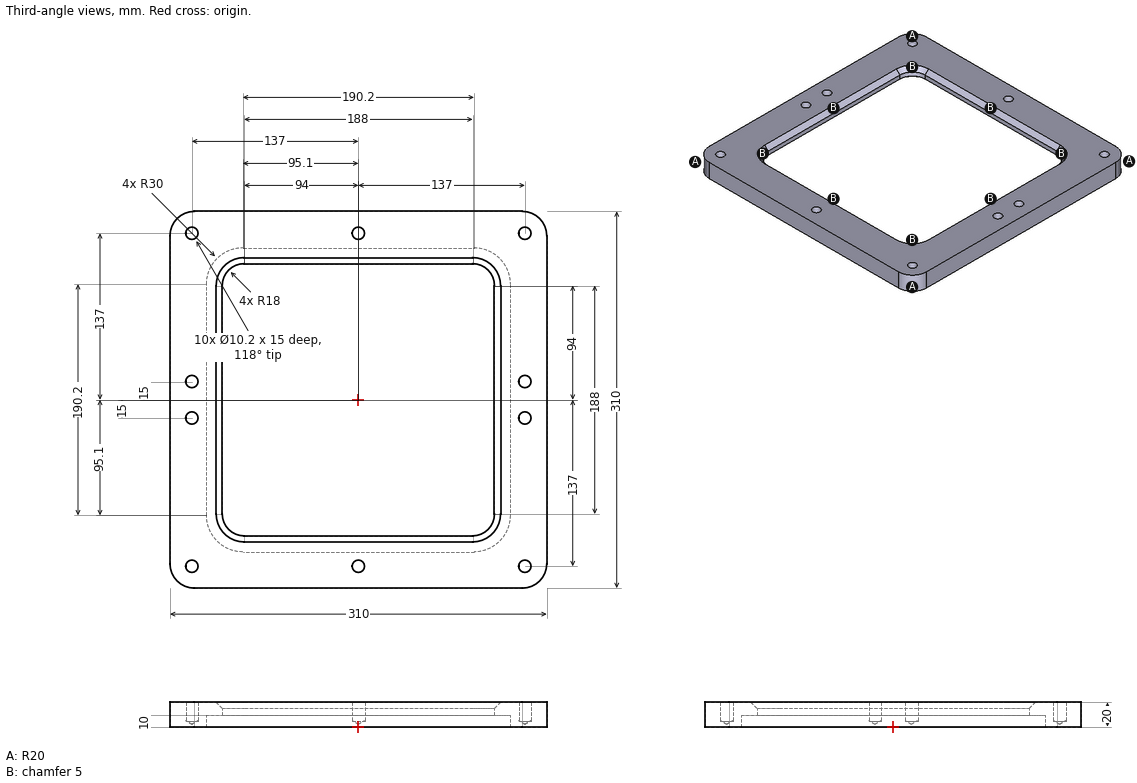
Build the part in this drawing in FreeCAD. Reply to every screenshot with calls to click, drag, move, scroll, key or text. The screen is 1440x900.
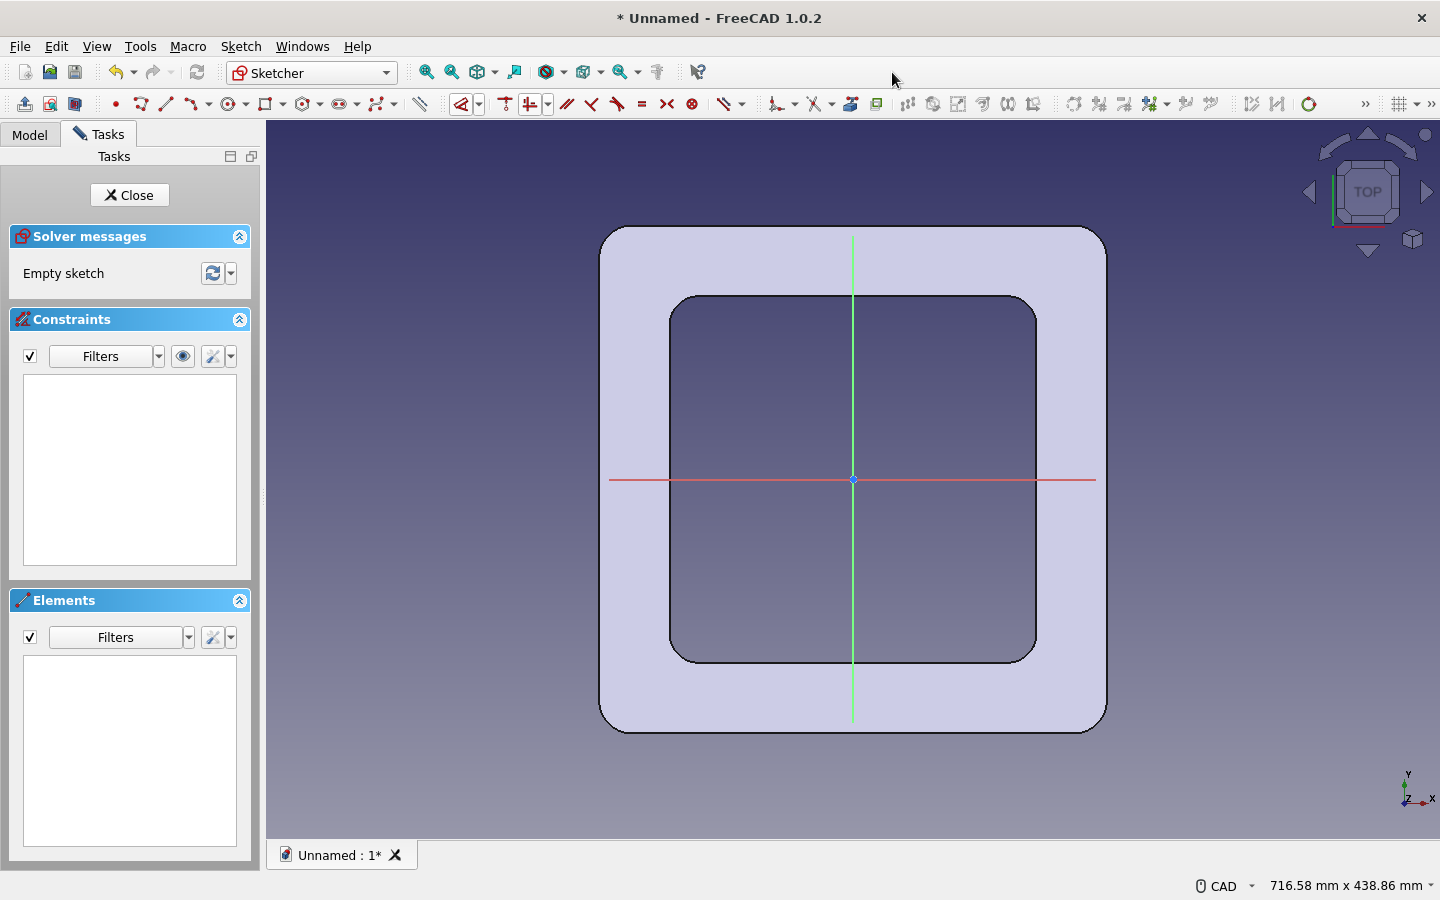
click(228, 104)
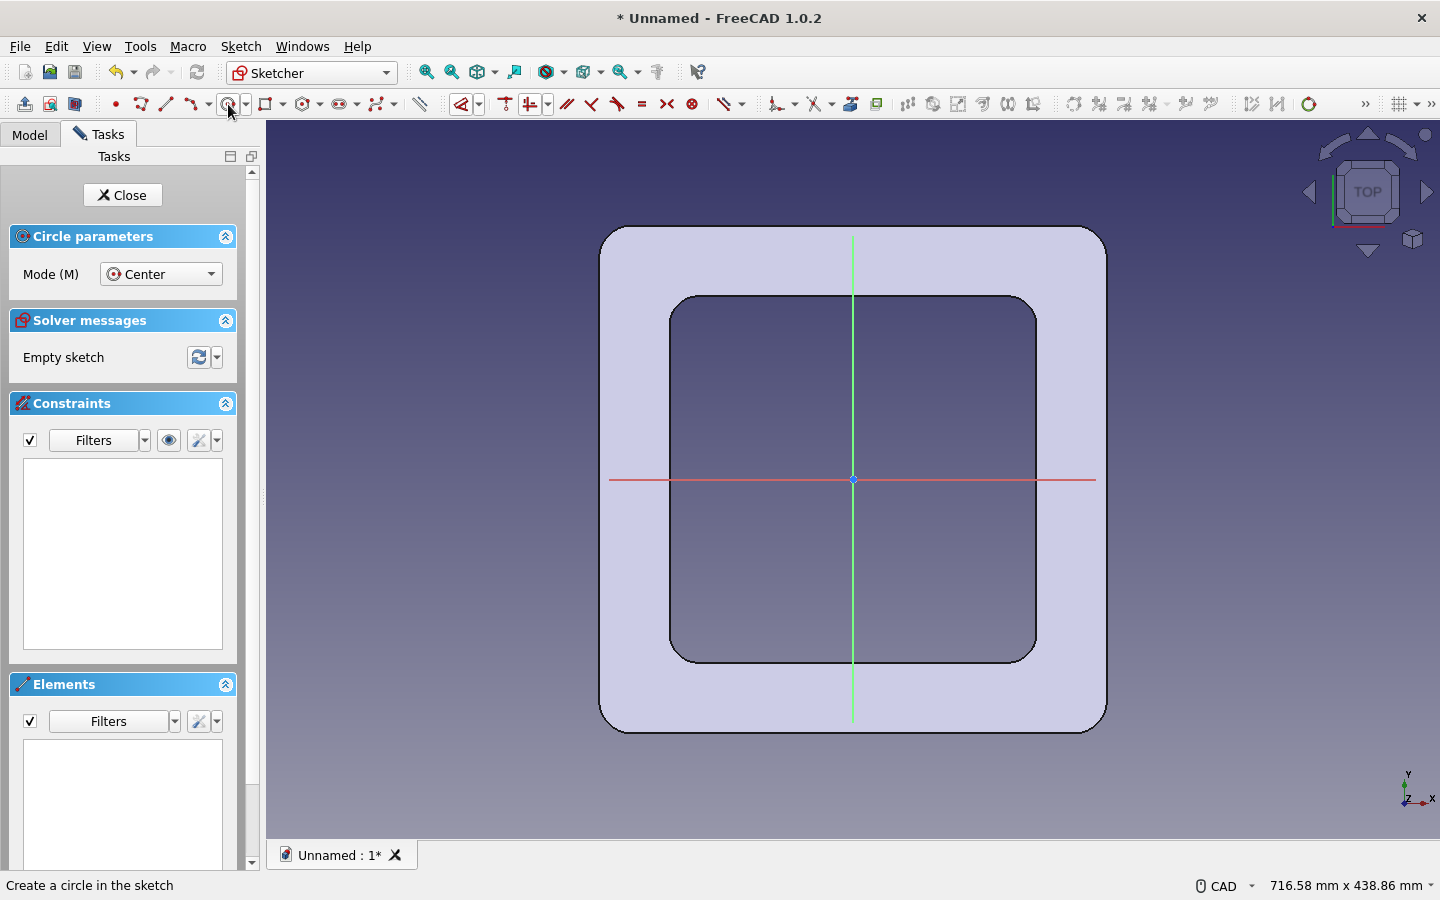
scroll(629, 255, up, 5)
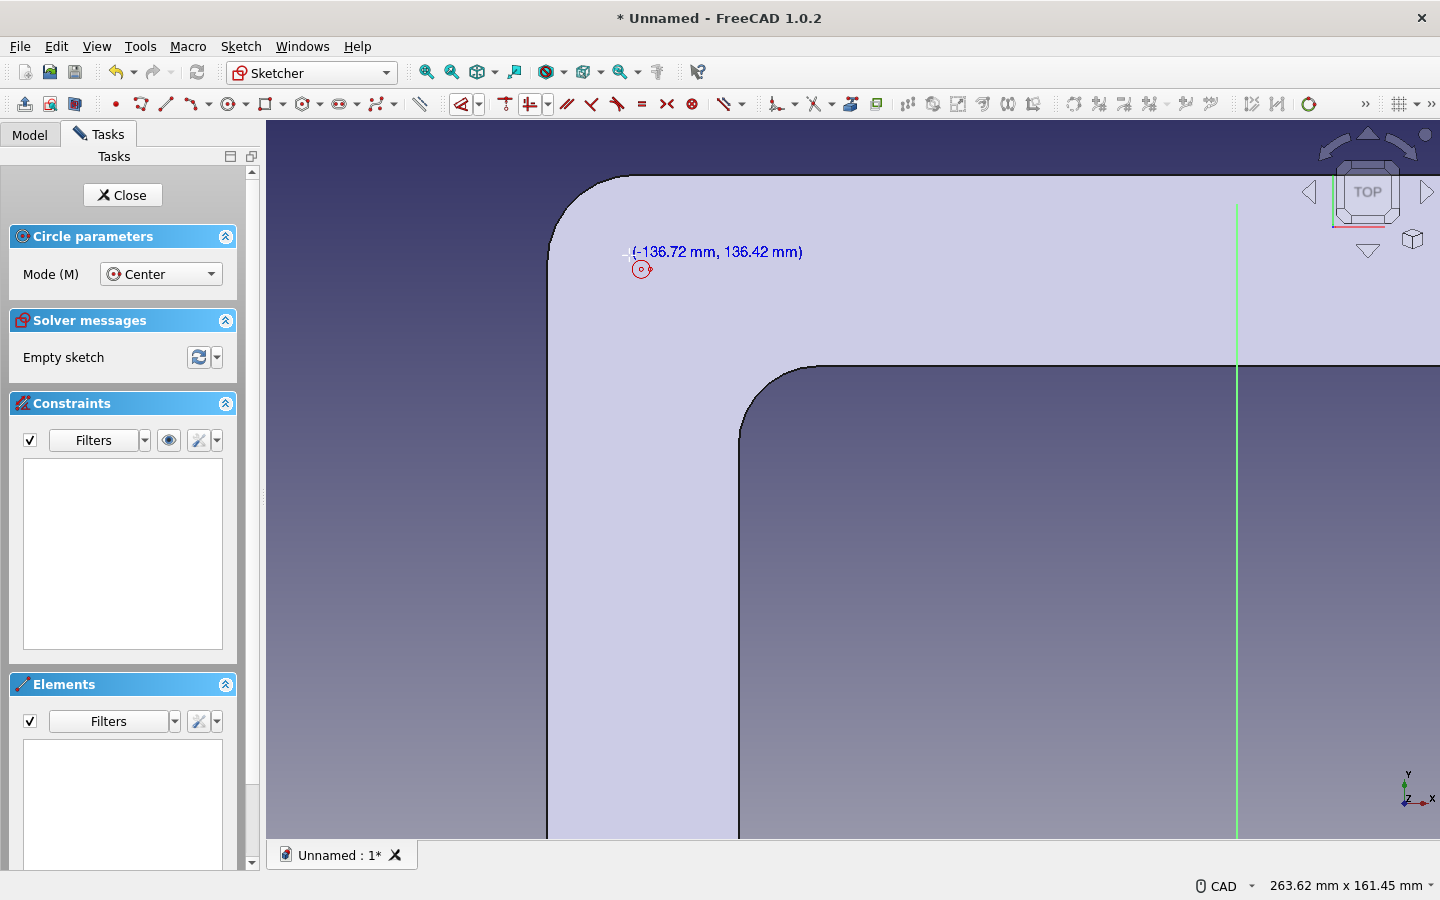
click(627, 255)
click(643, 239)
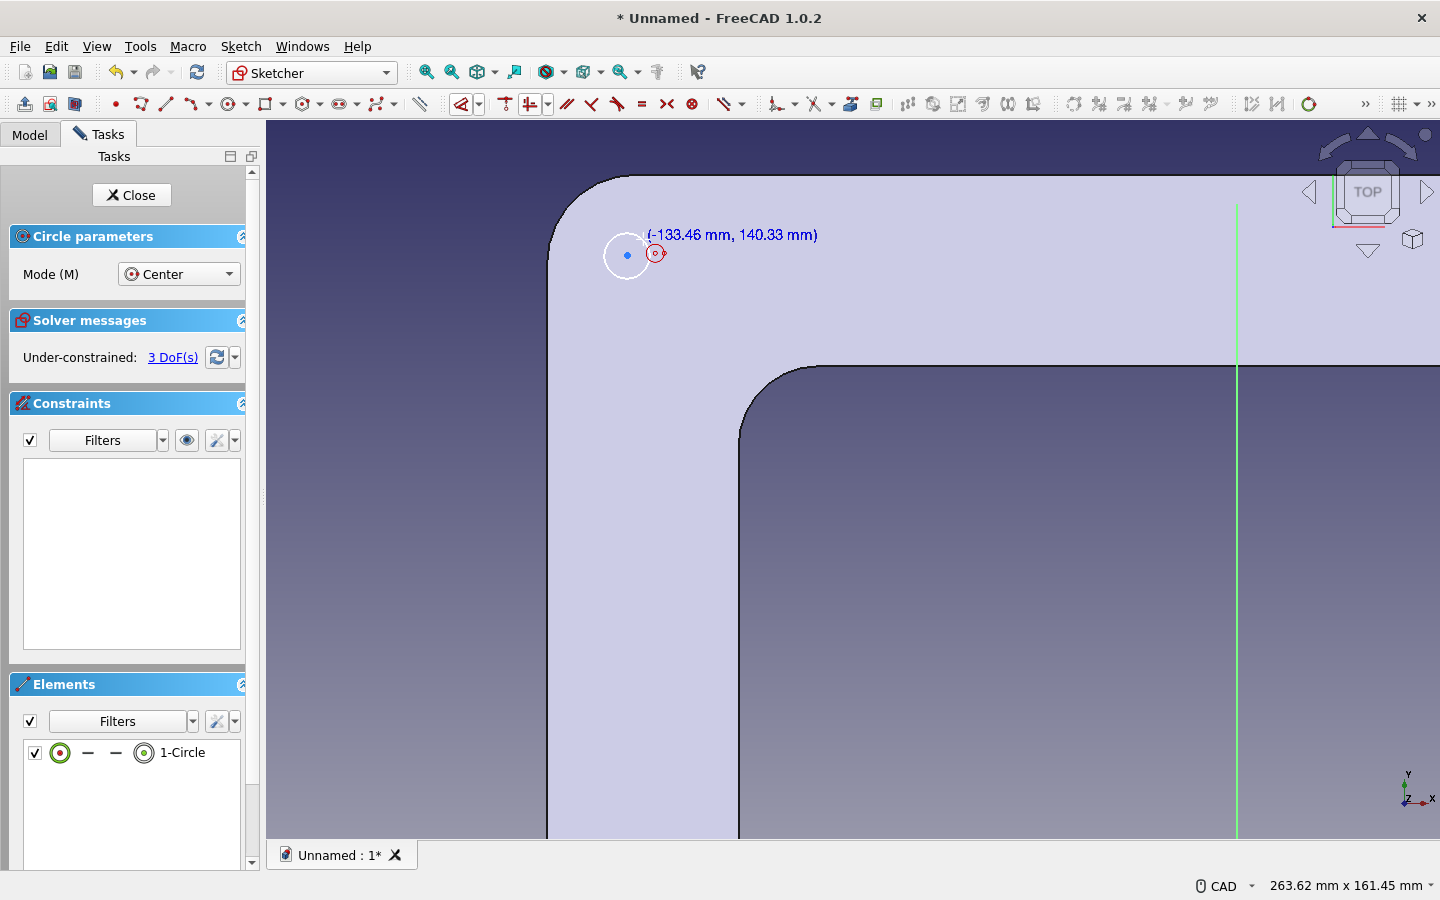
scroll(521, 255, down, 5)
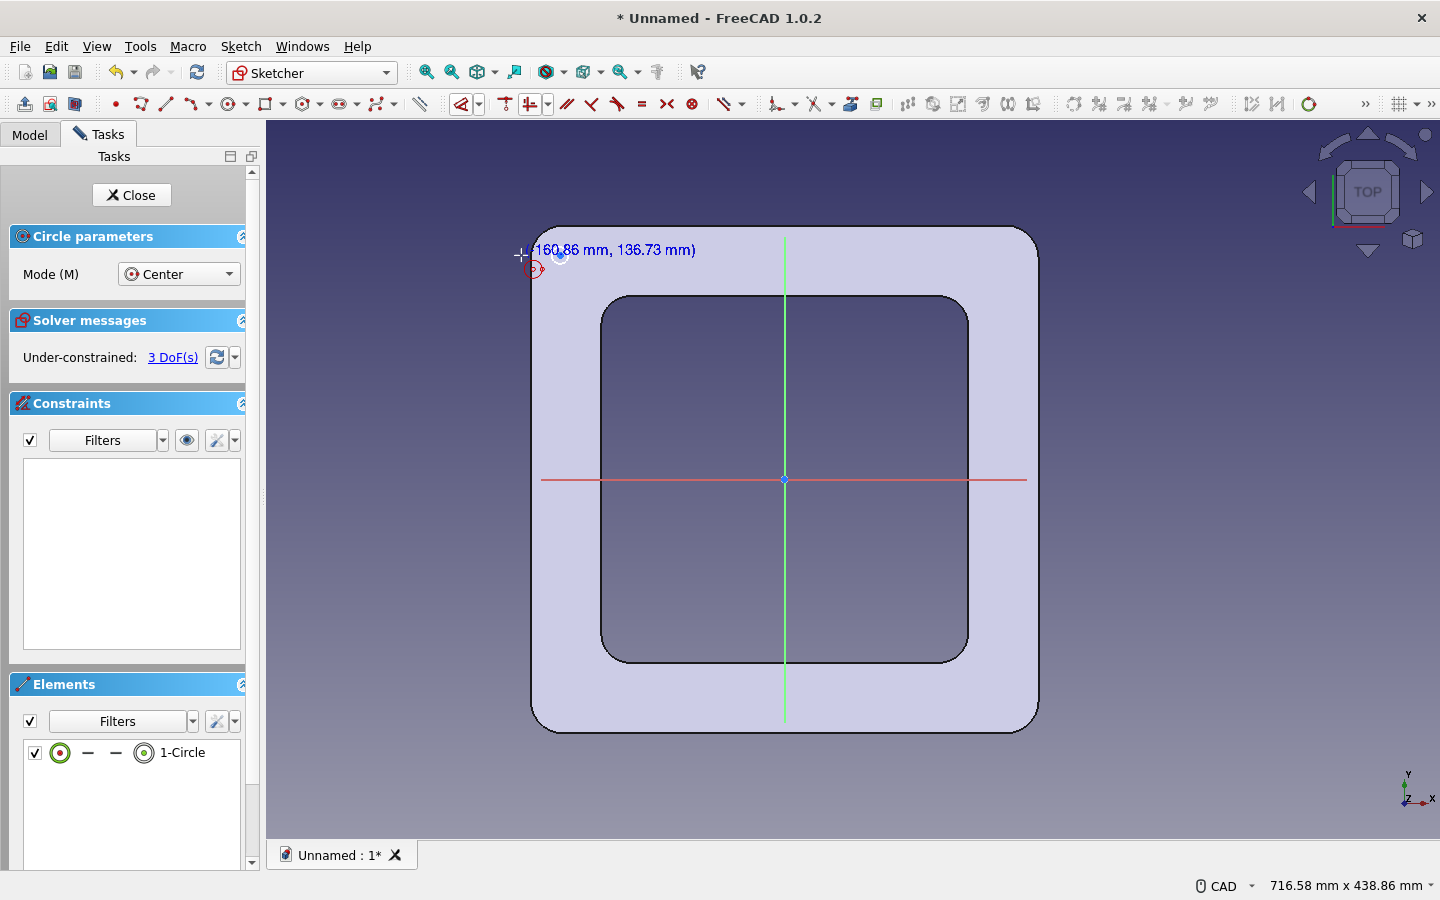
scroll(1009, 255, up, 5)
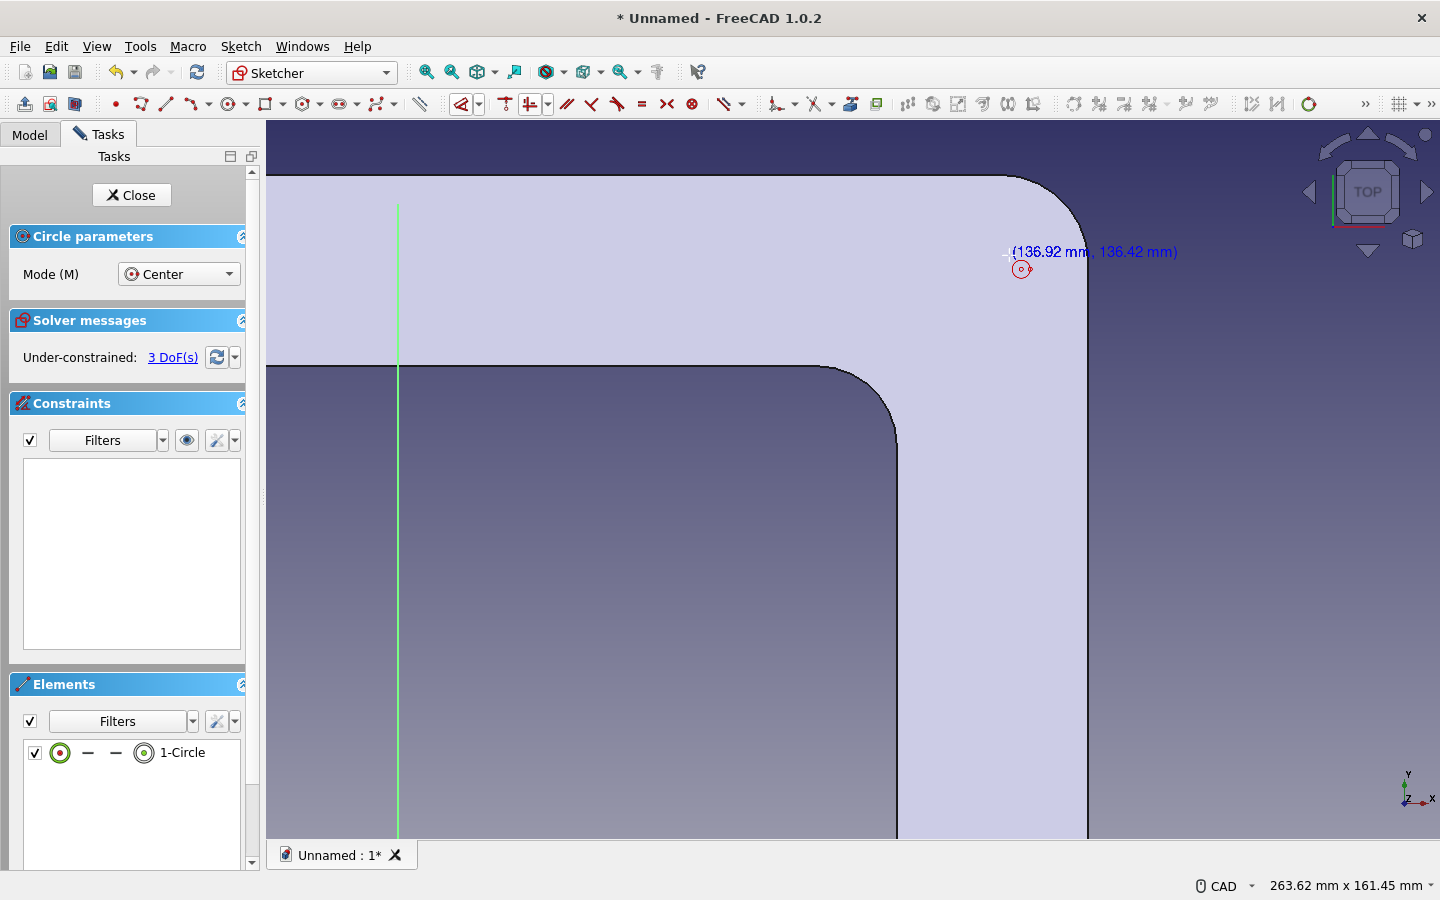
click(1008, 255)
click(1024, 239)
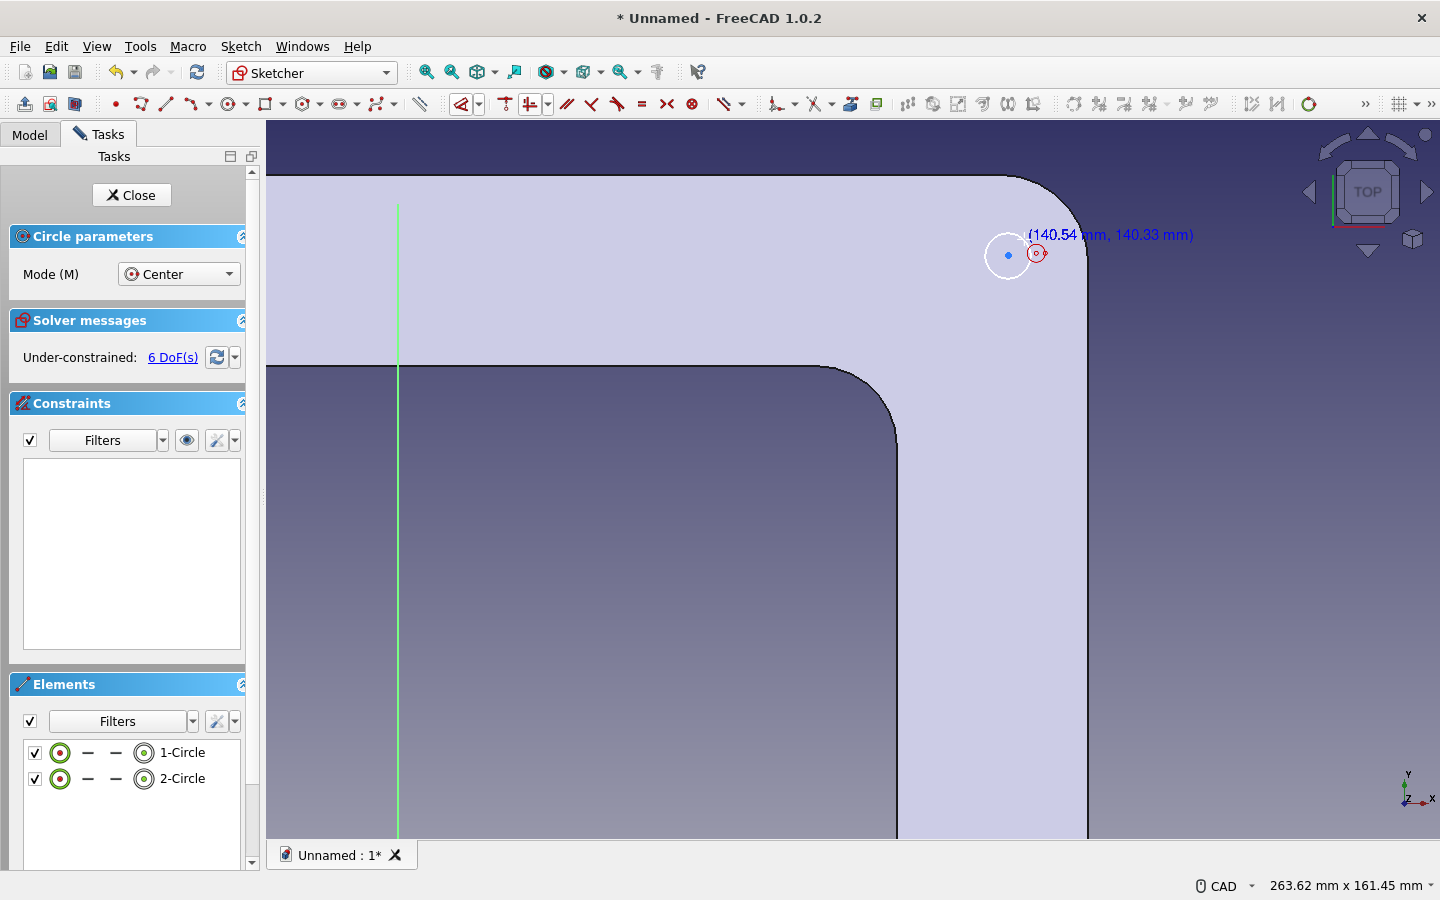
scroll(1009, 255, down, 5)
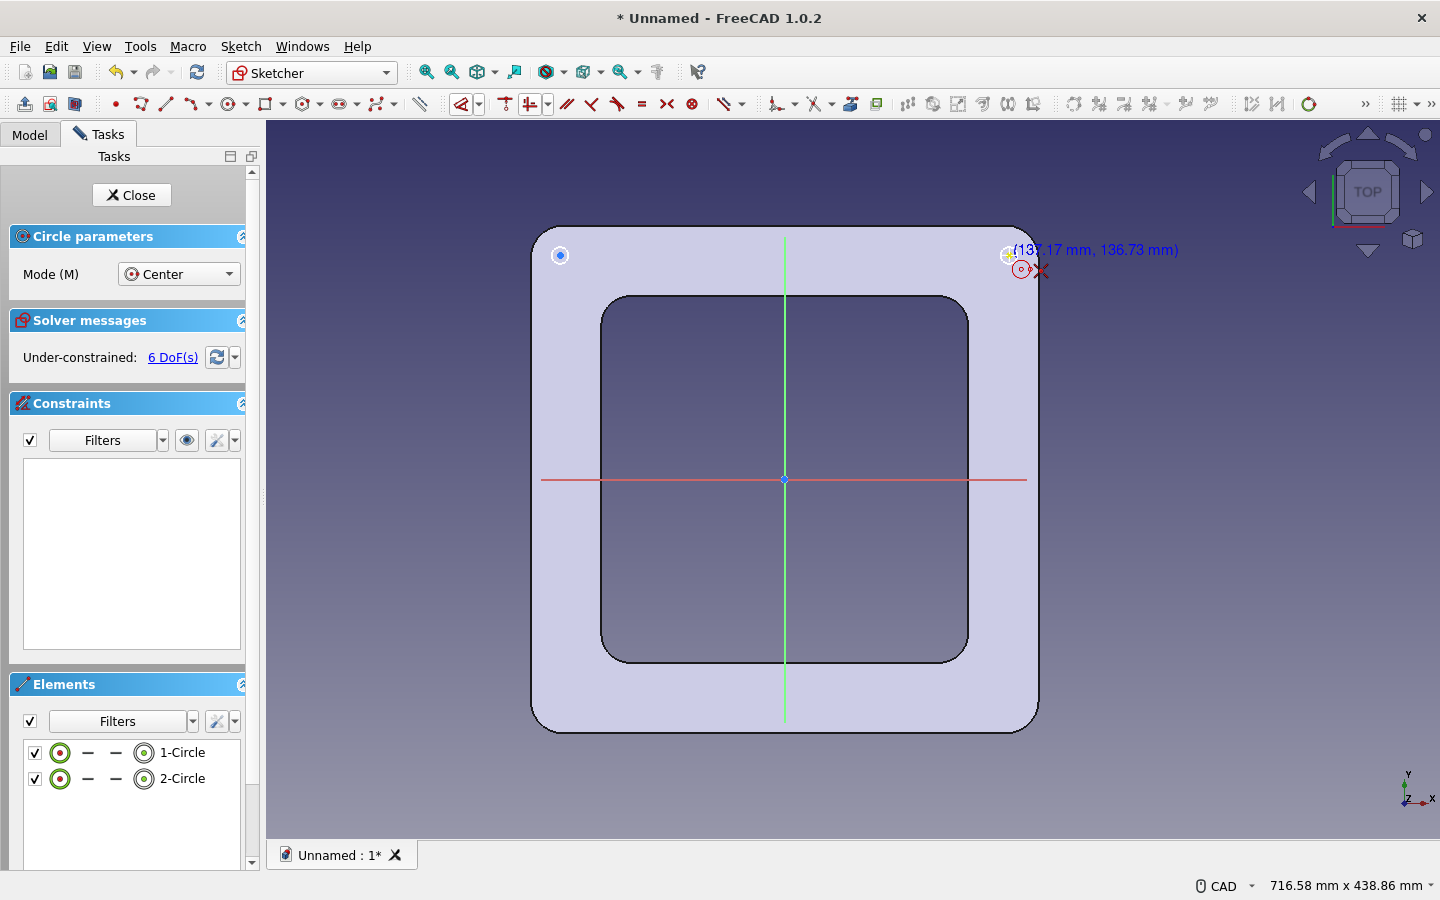
scroll(1009, 704, up, 5)